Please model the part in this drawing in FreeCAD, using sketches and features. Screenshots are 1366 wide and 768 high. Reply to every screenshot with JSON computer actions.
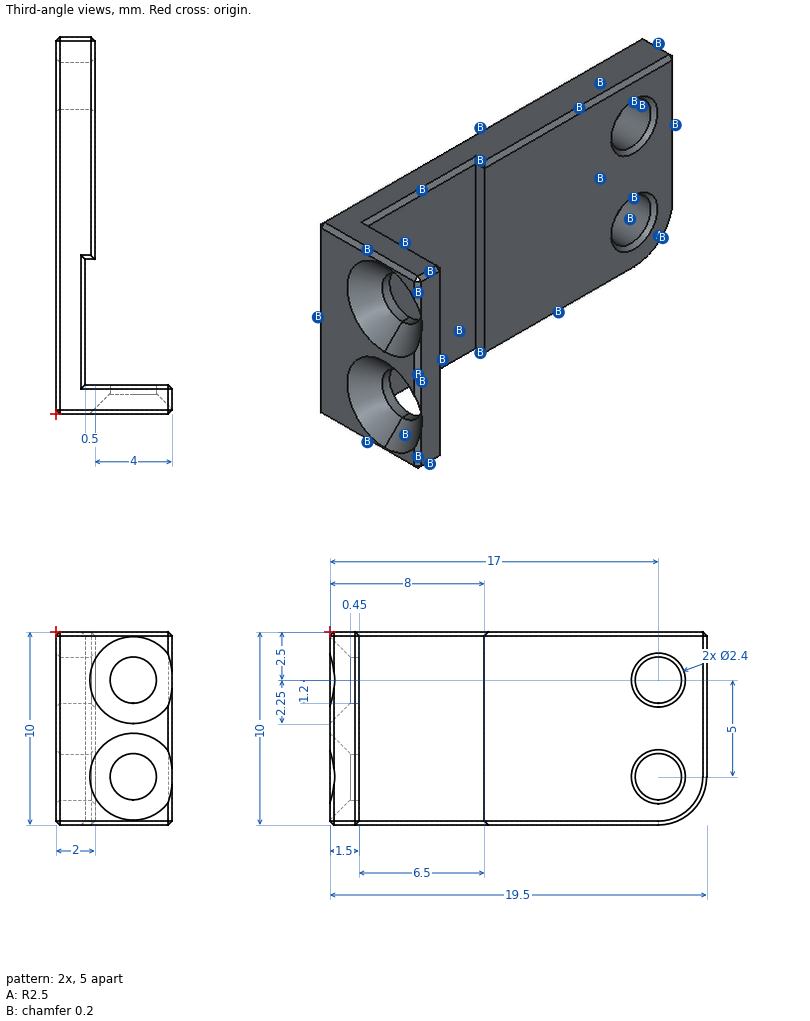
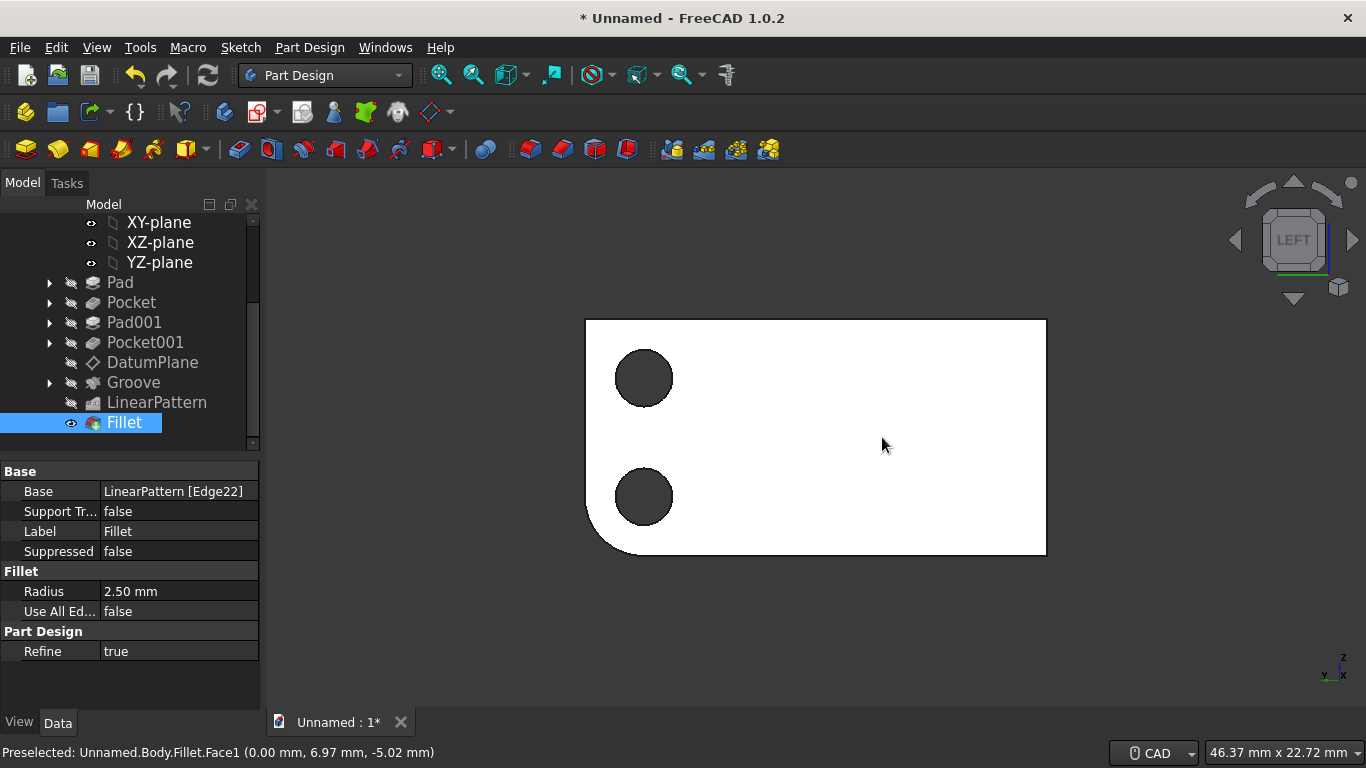
{"action": "scroll", "coordinate": [858, 555], "scroll_direction": "up", "scroll_amount": 7}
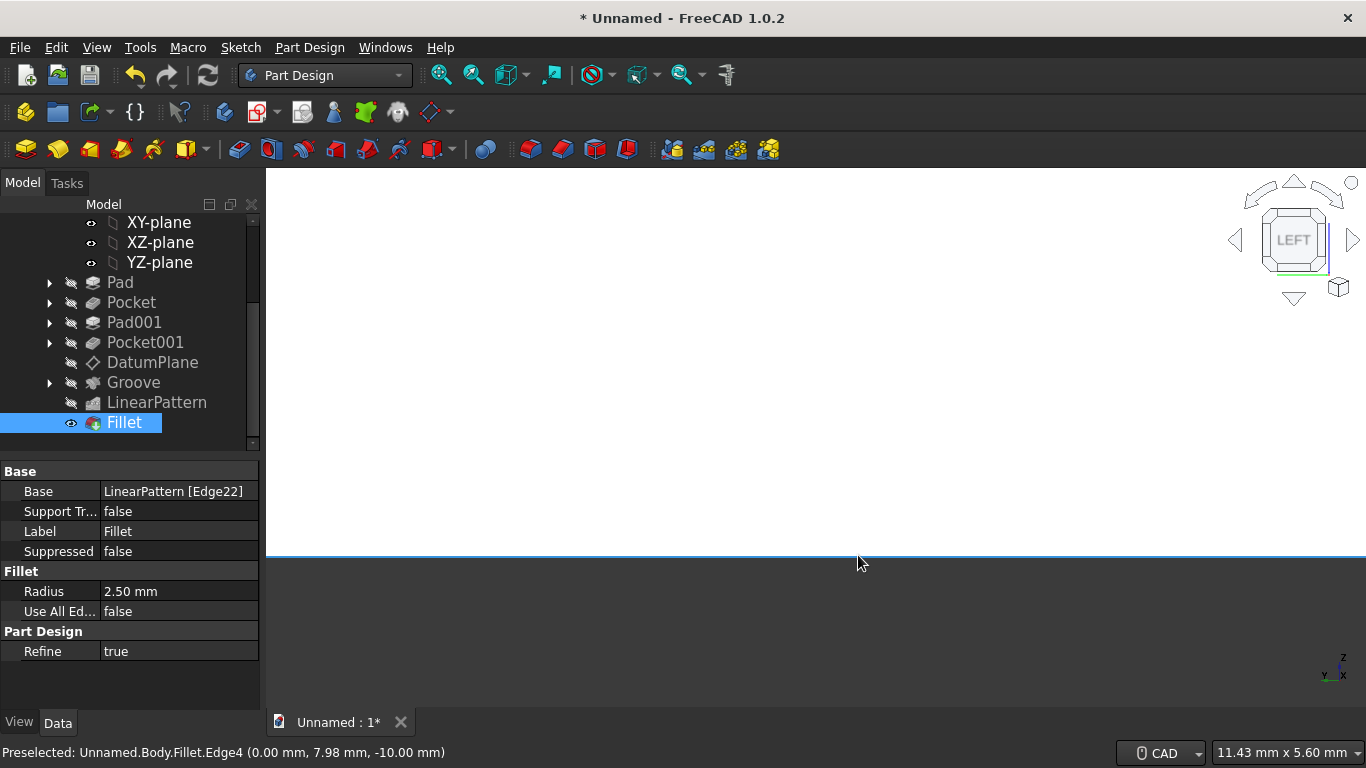
{"action": "left_click", "coordinate": [442, 76]}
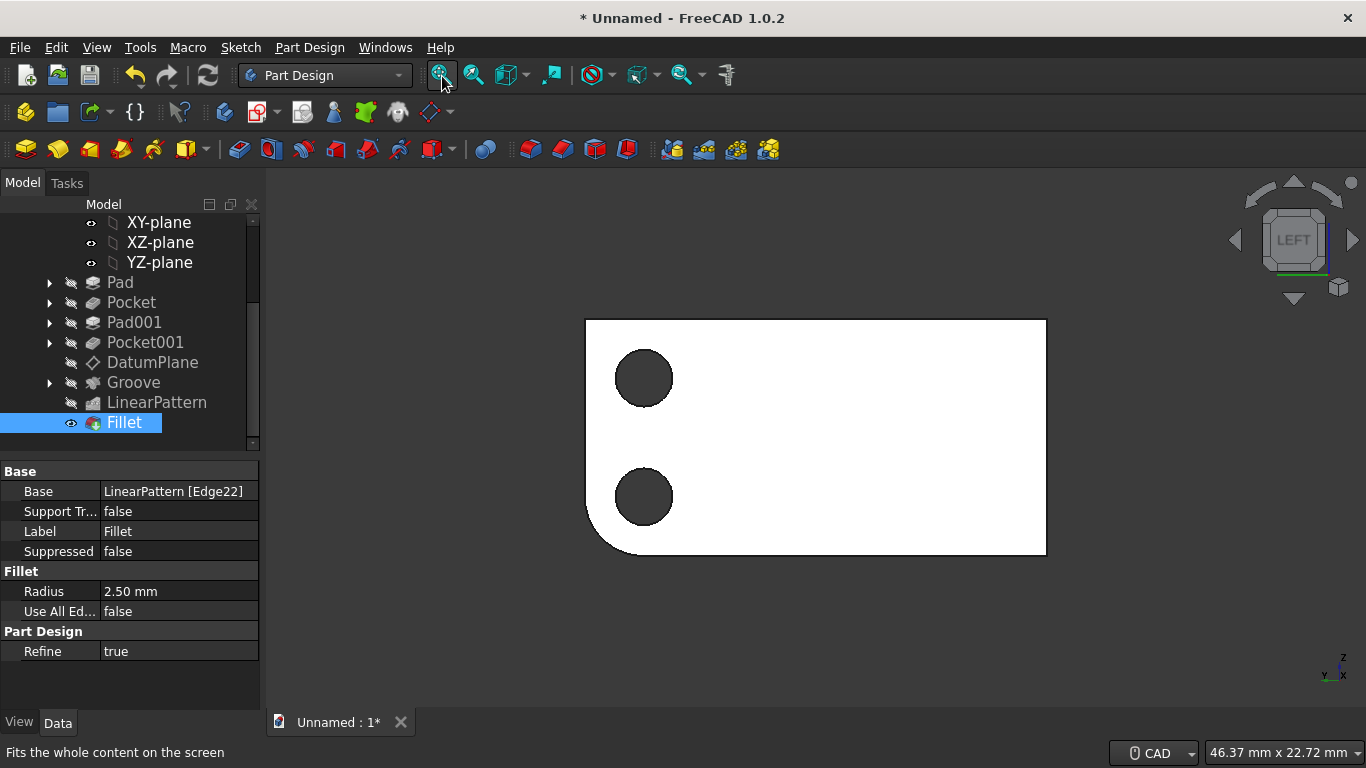
{"action": "key", "text": "v 3"}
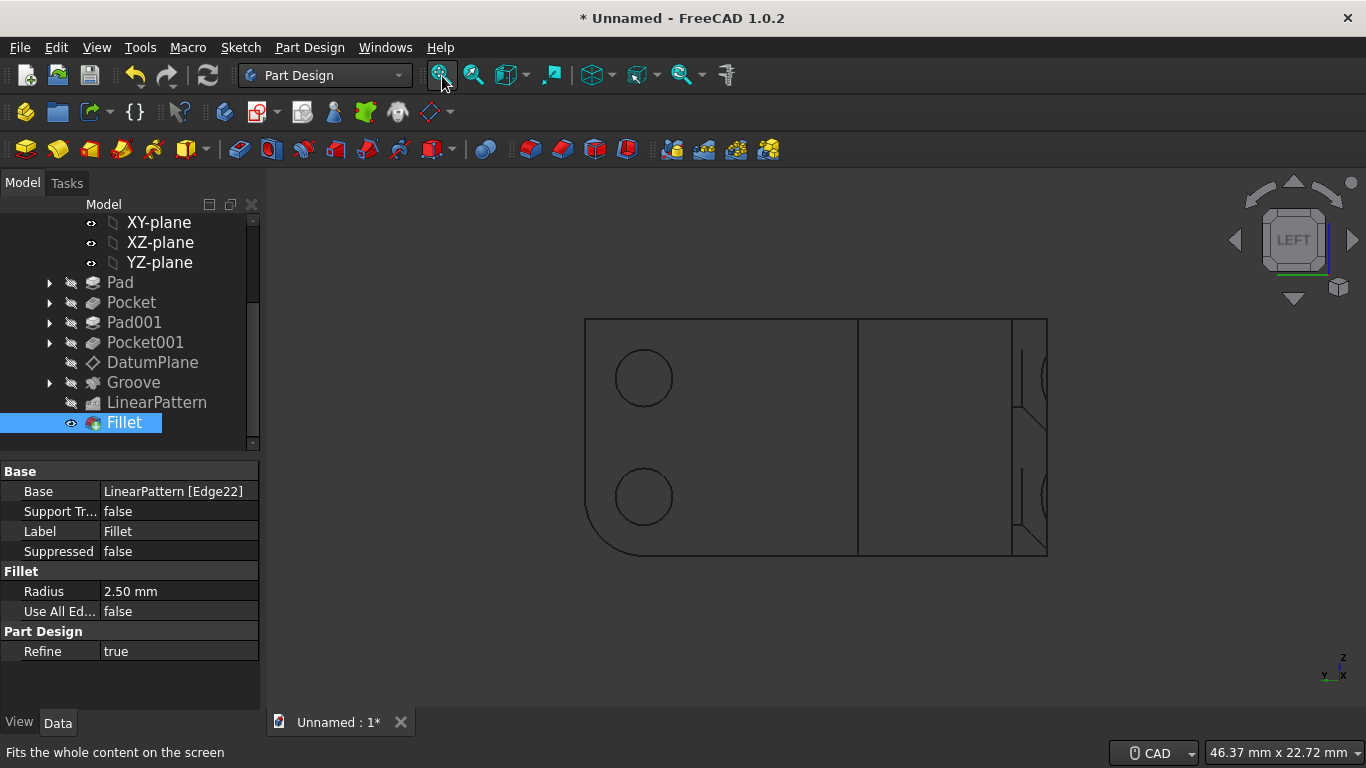
{"action": "key", "text": "0"}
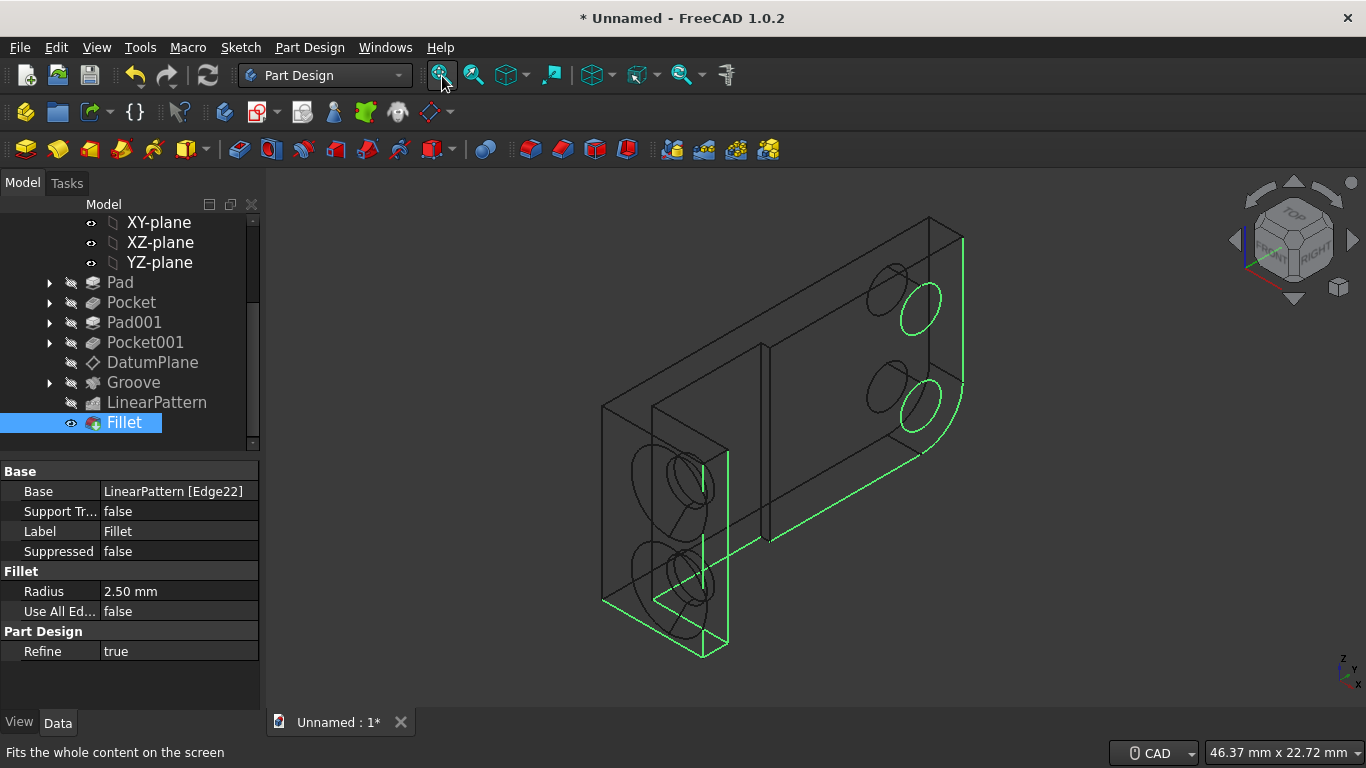
{"action": "scroll", "coordinate": [766, 538], "scroll_direction": "up", "scroll_amount": 7}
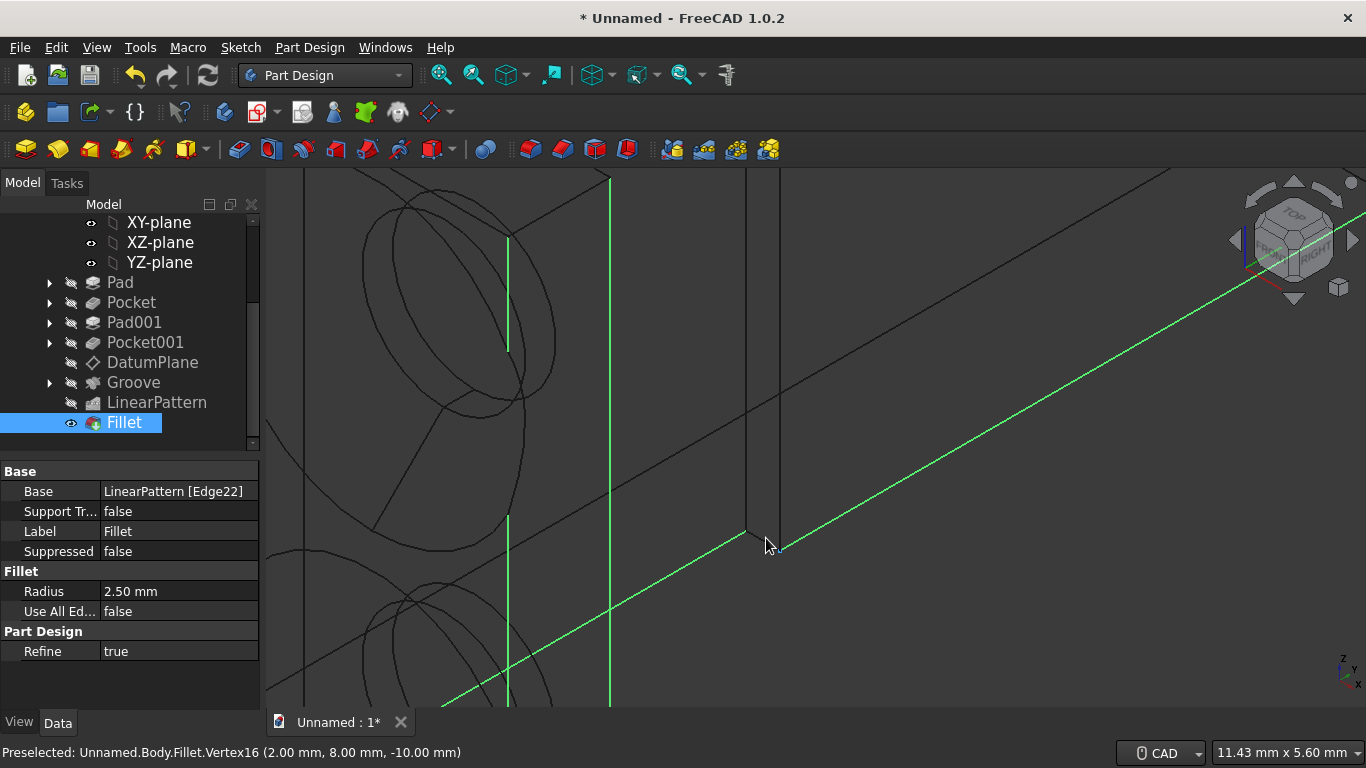
{"action": "left_click", "coordinate": [763, 540], "text": "ctrl"}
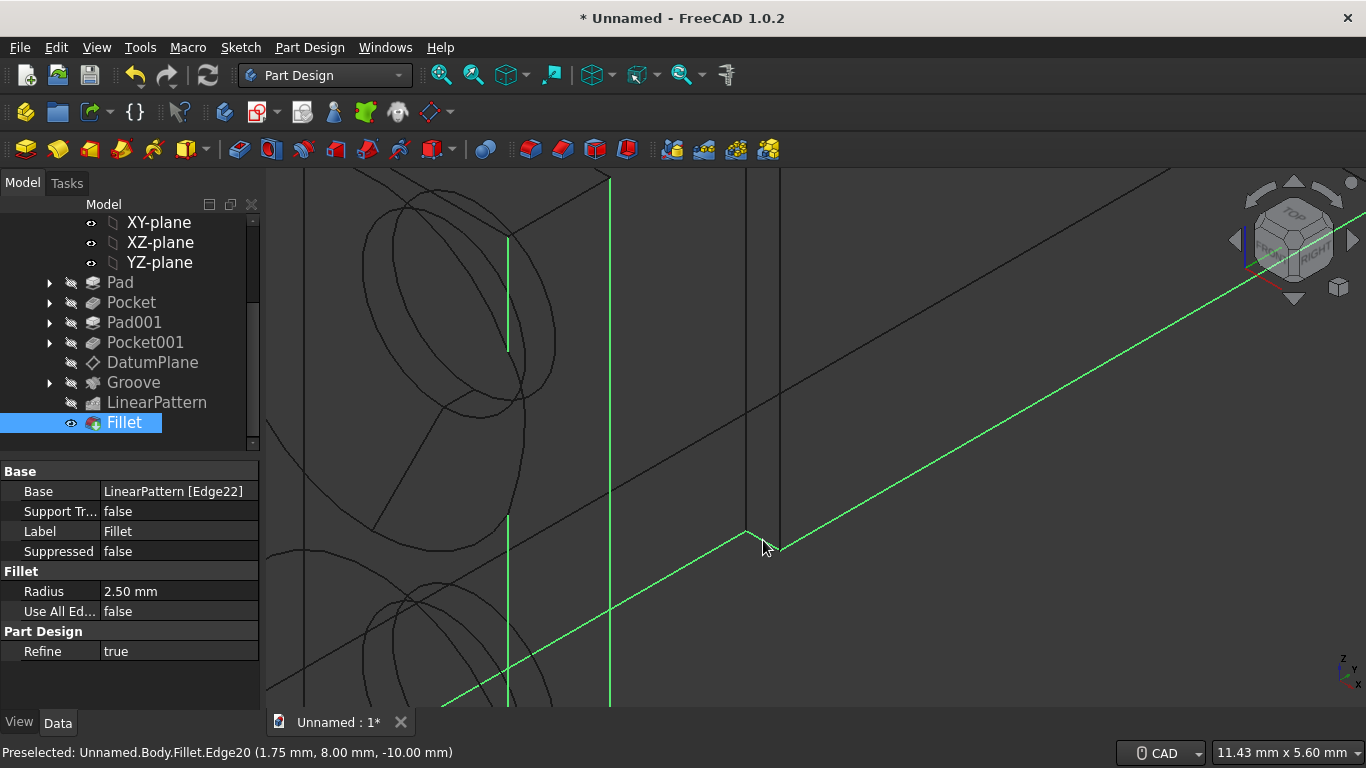
{"action": "key", "text": "v 1"}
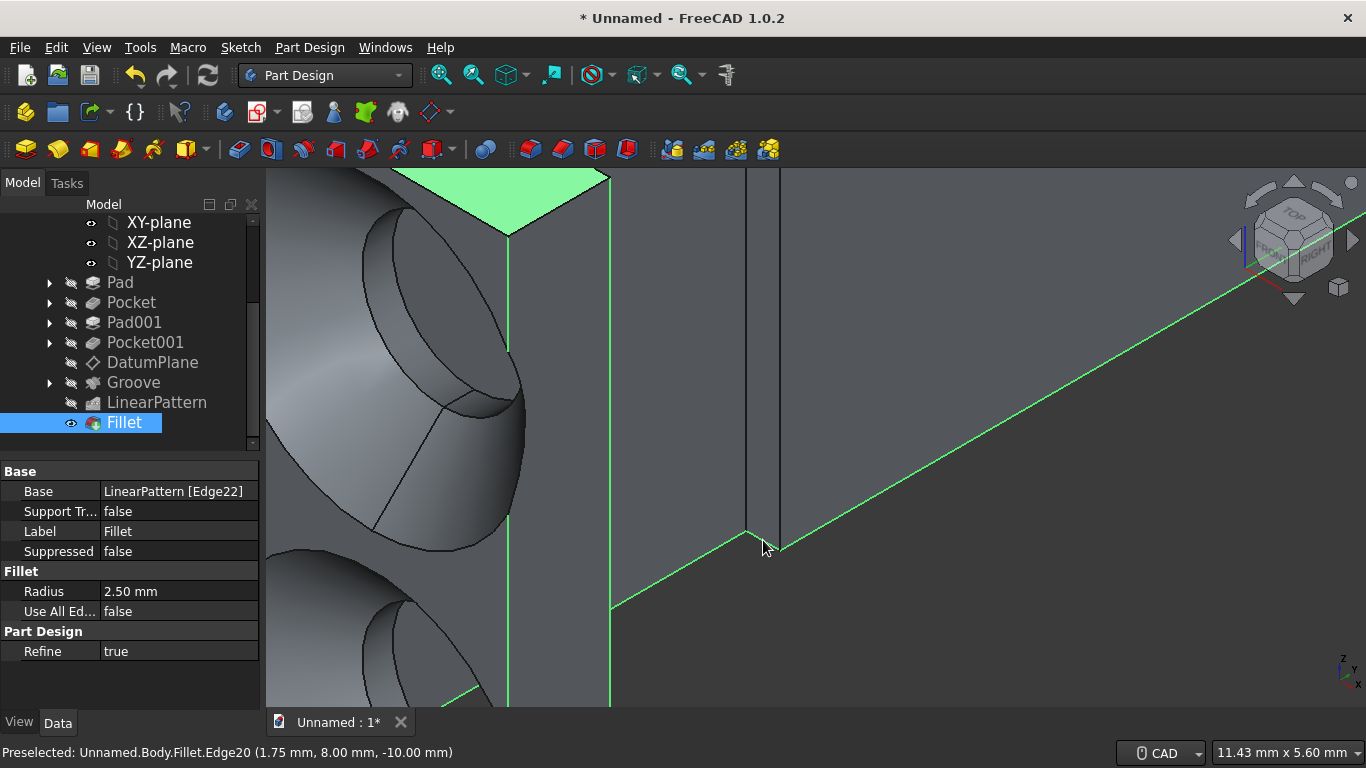
{"action": "left_click", "coordinate": [564, 150]}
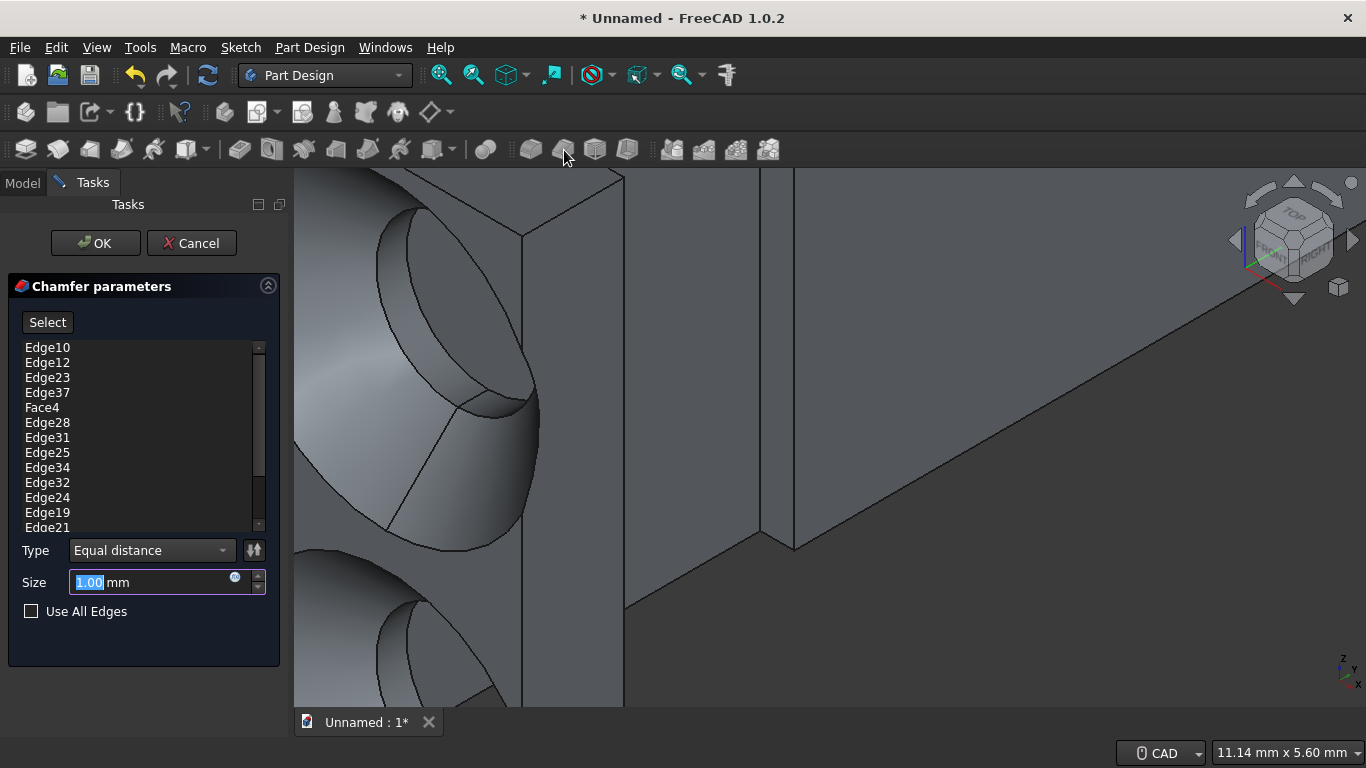
{"action": "type", "text": "0.2"}
{"action": "key", "text": "Tab"}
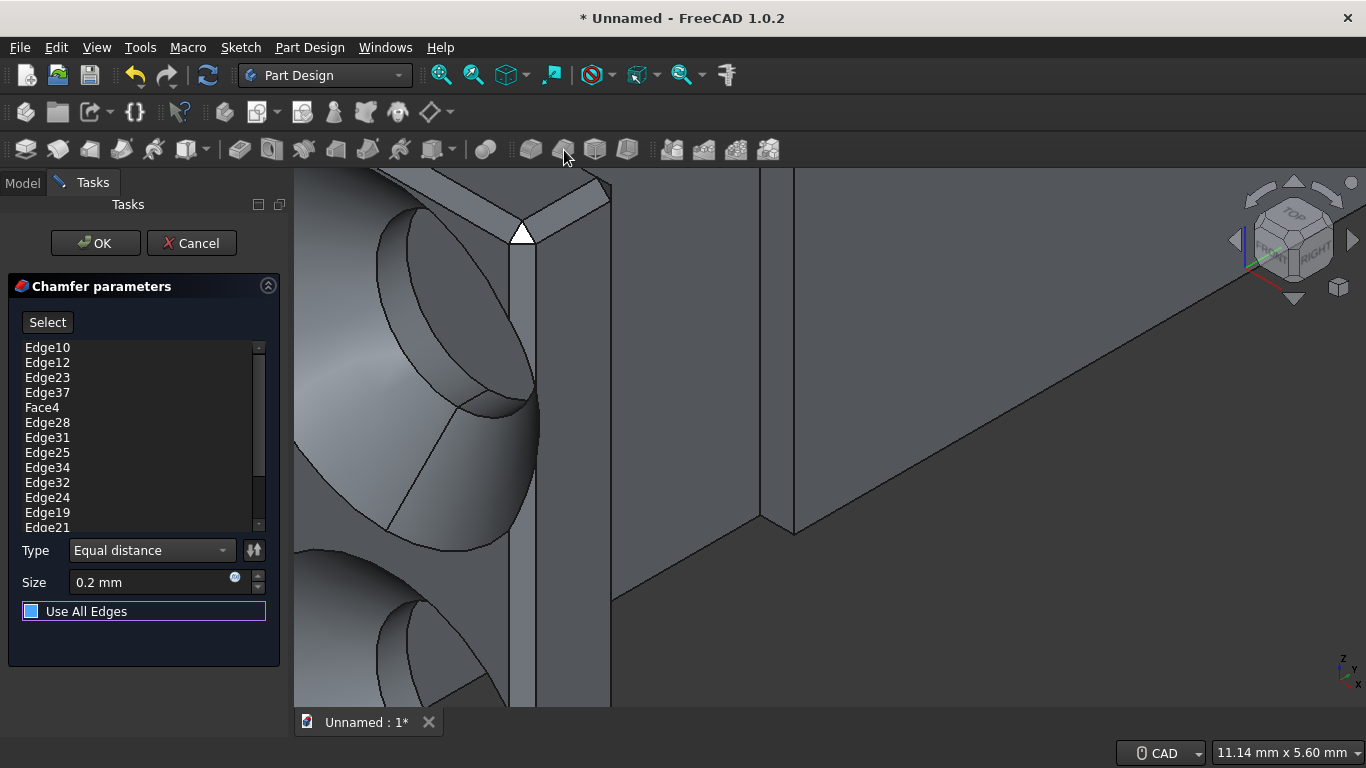
{"action": "left_click", "coordinate": [96, 243]}